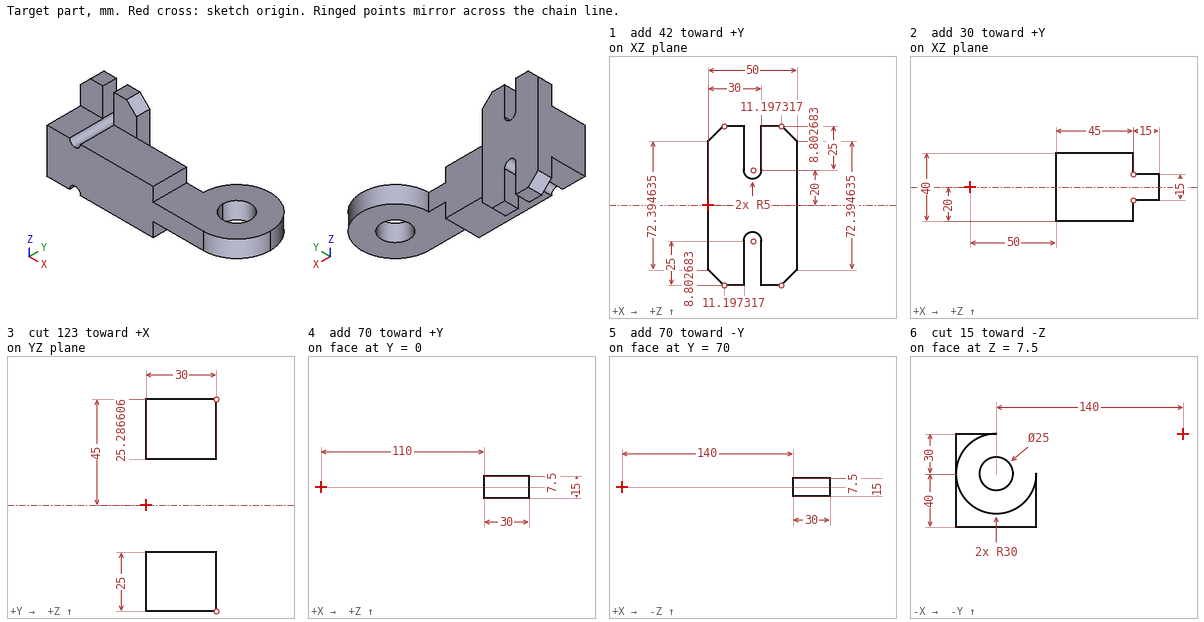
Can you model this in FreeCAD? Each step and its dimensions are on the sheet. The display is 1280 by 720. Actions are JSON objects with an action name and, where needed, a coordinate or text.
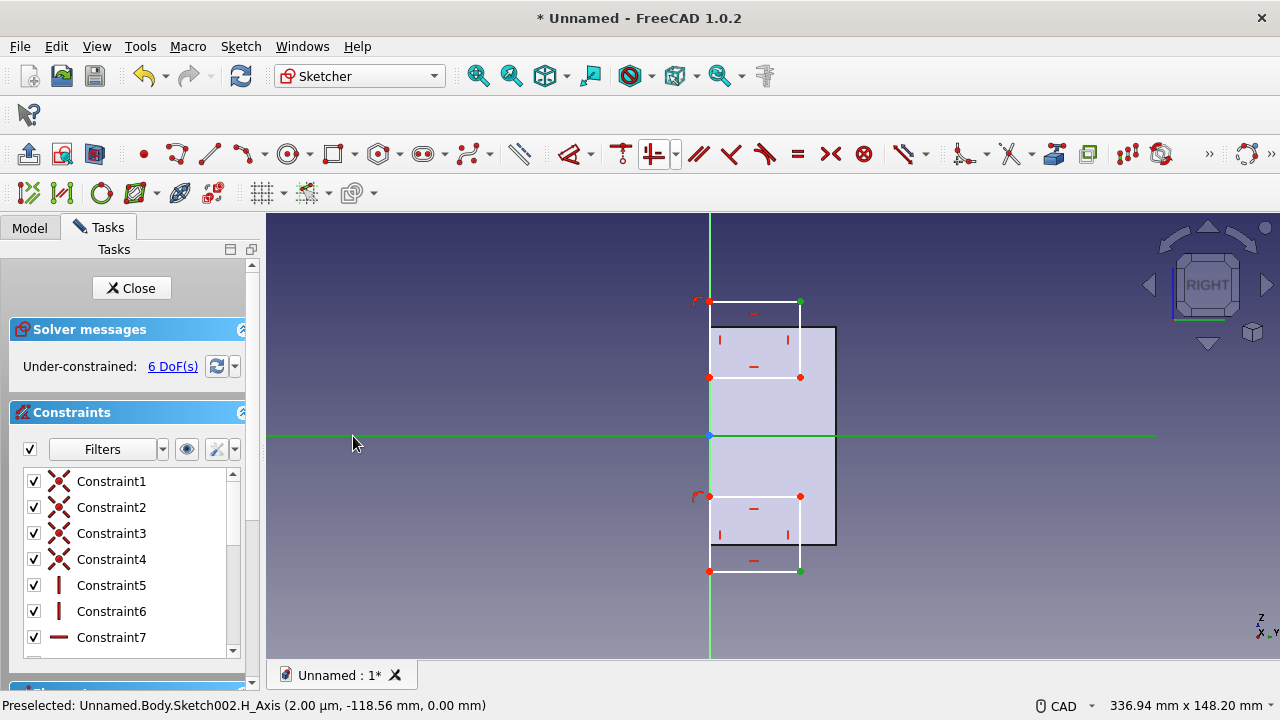
{"action": "left_click", "coordinate": [831, 154]}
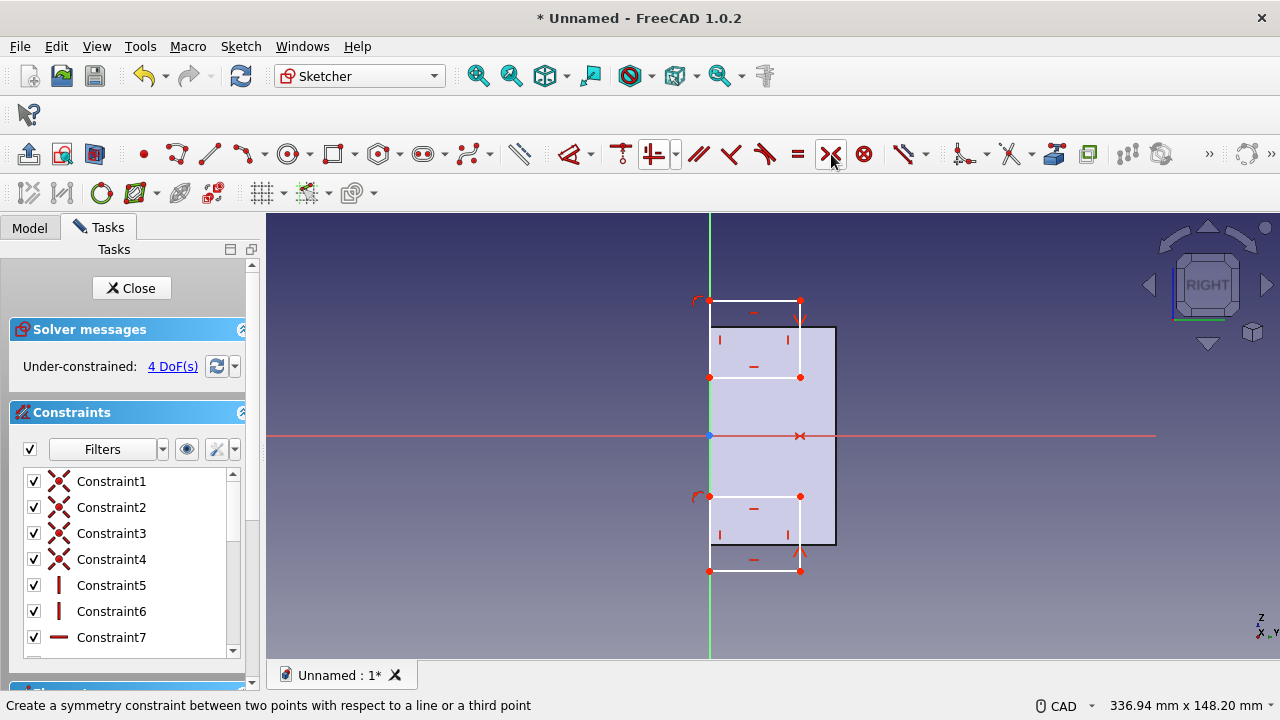
{"action": "left_click", "coordinate": [568, 154]}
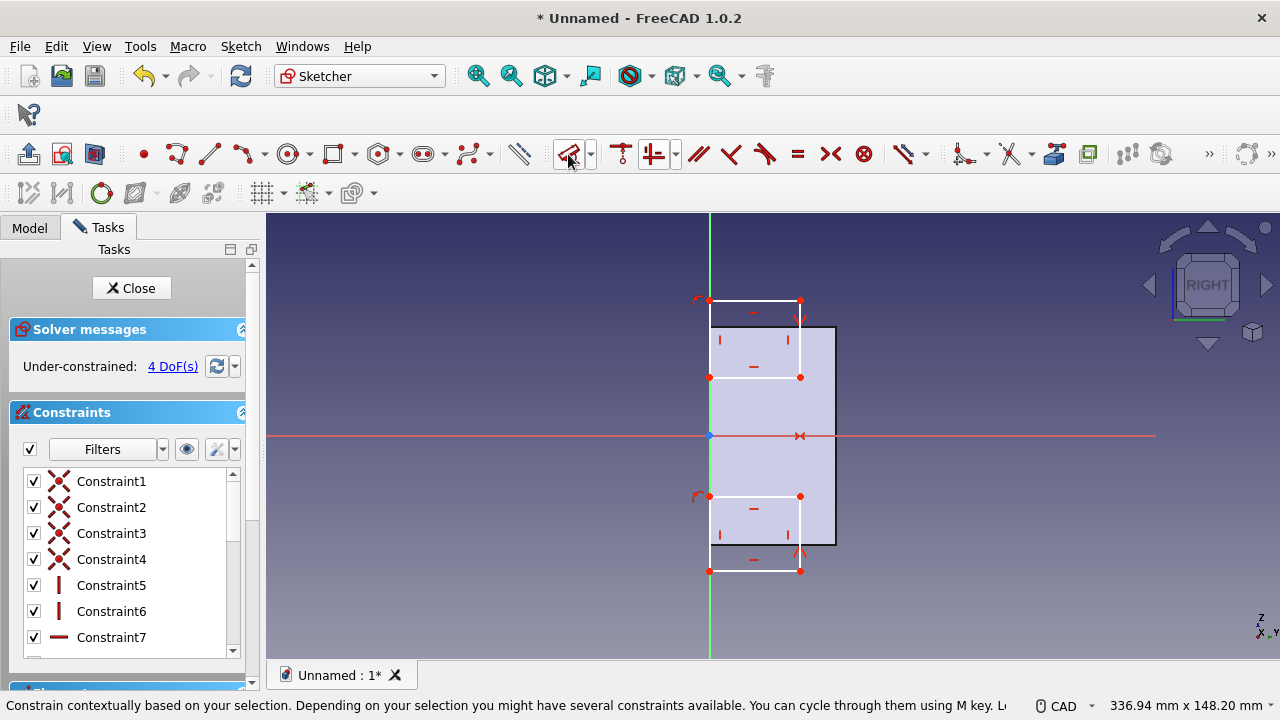
{"action": "left_click", "coordinate": [737, 378]}
{"action": "left_click", "coordinate": [755, 344]}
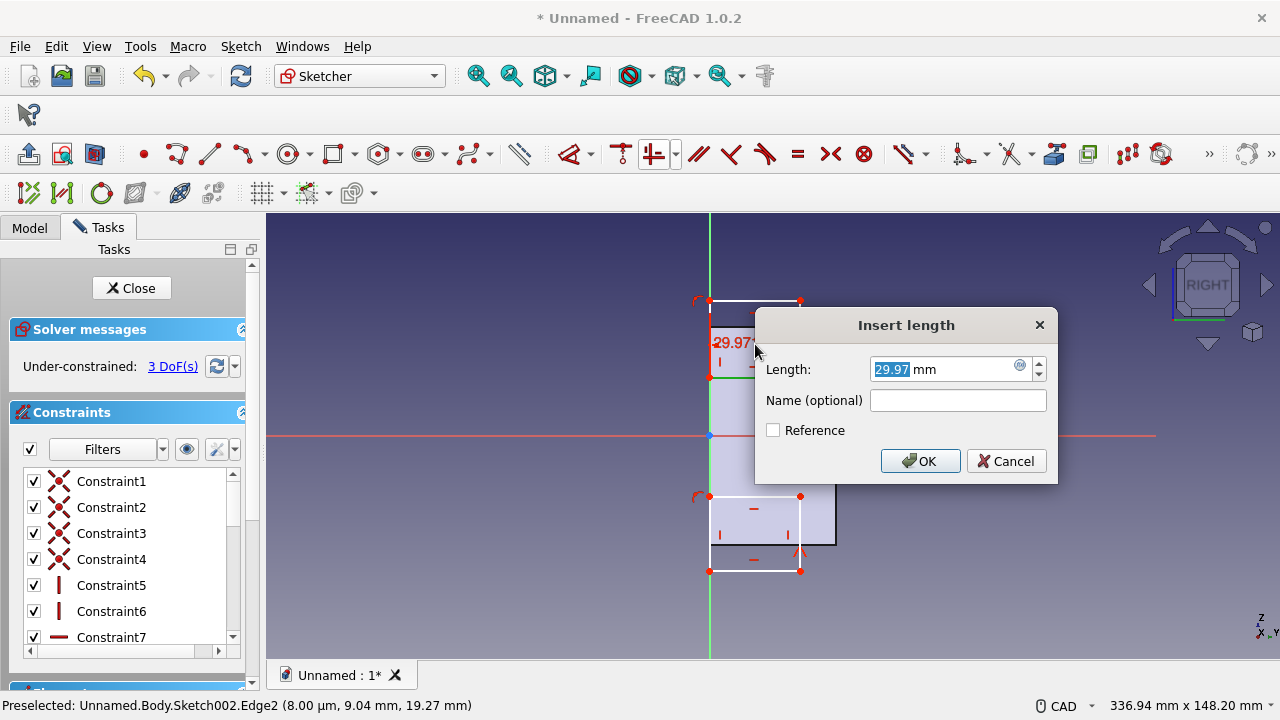
{"action": "type", "text": "30"}
{"action": "key", "text": "Return"}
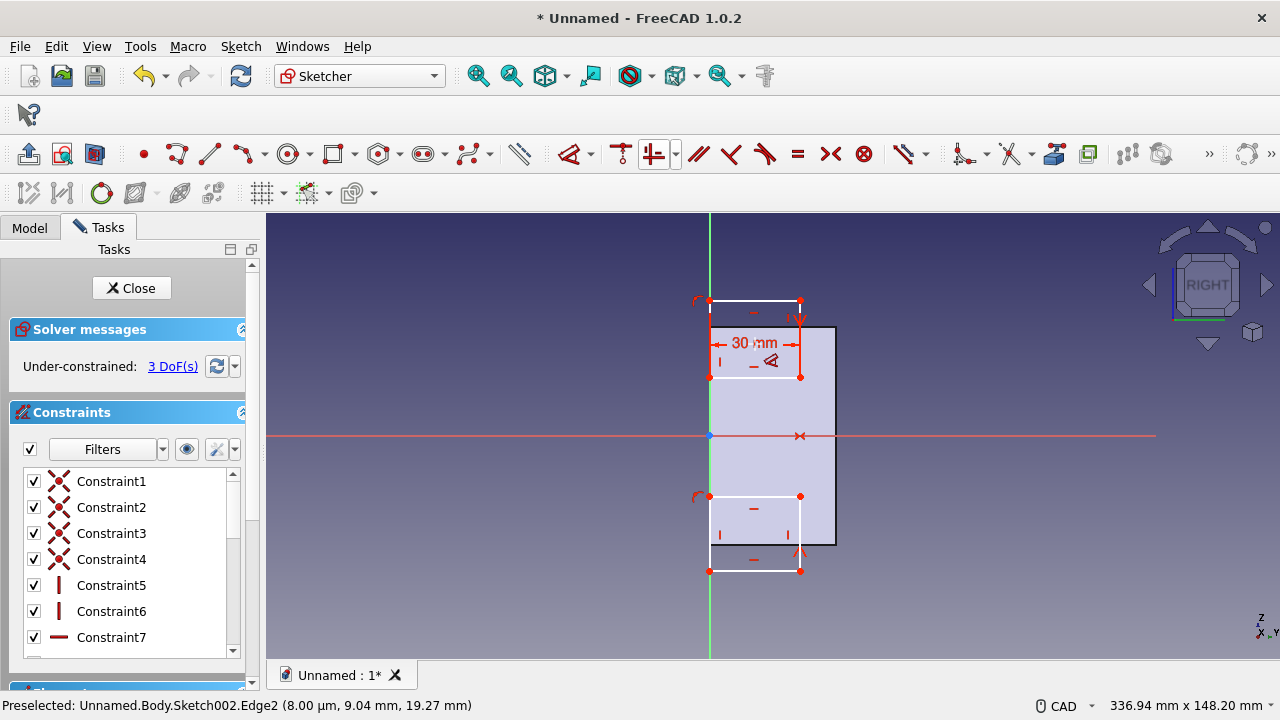
{"action": "left_click", "coordinate": [710, 519]}
{"action": "left_click", "coordinate": [676, 534]}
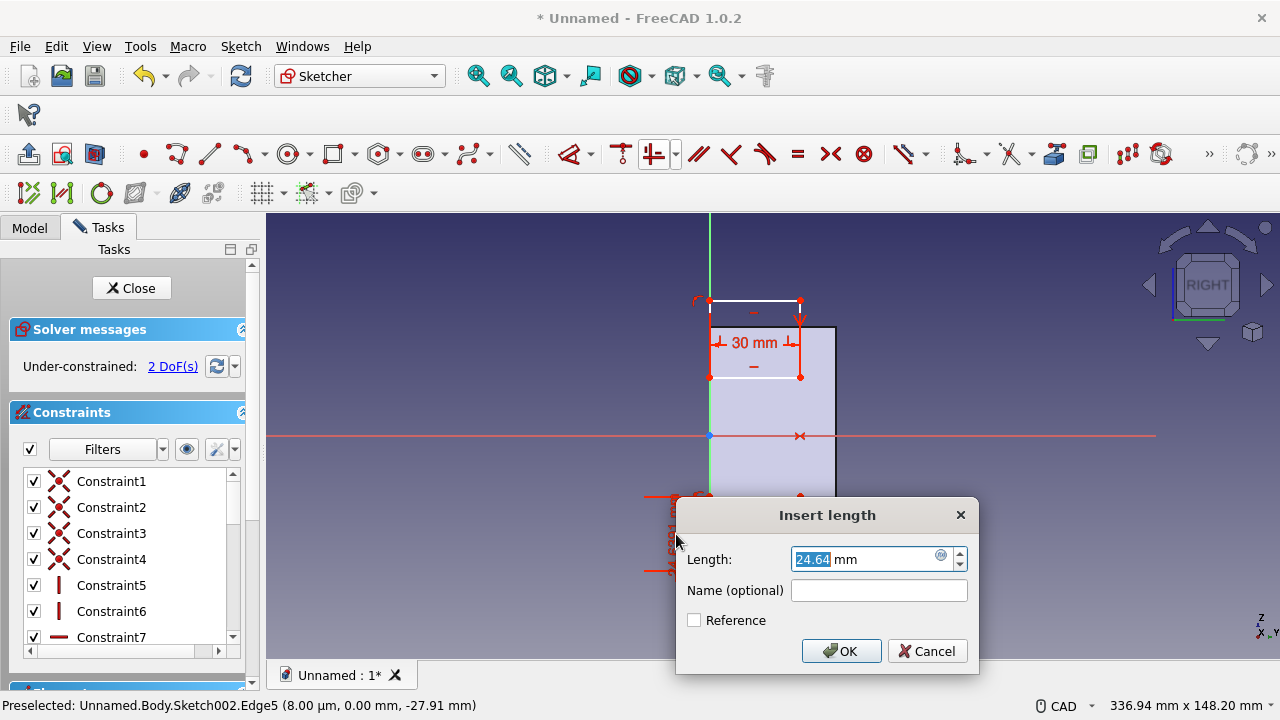
{"action": "type", "text": "25"}
{"action": "key", "text": "Return"}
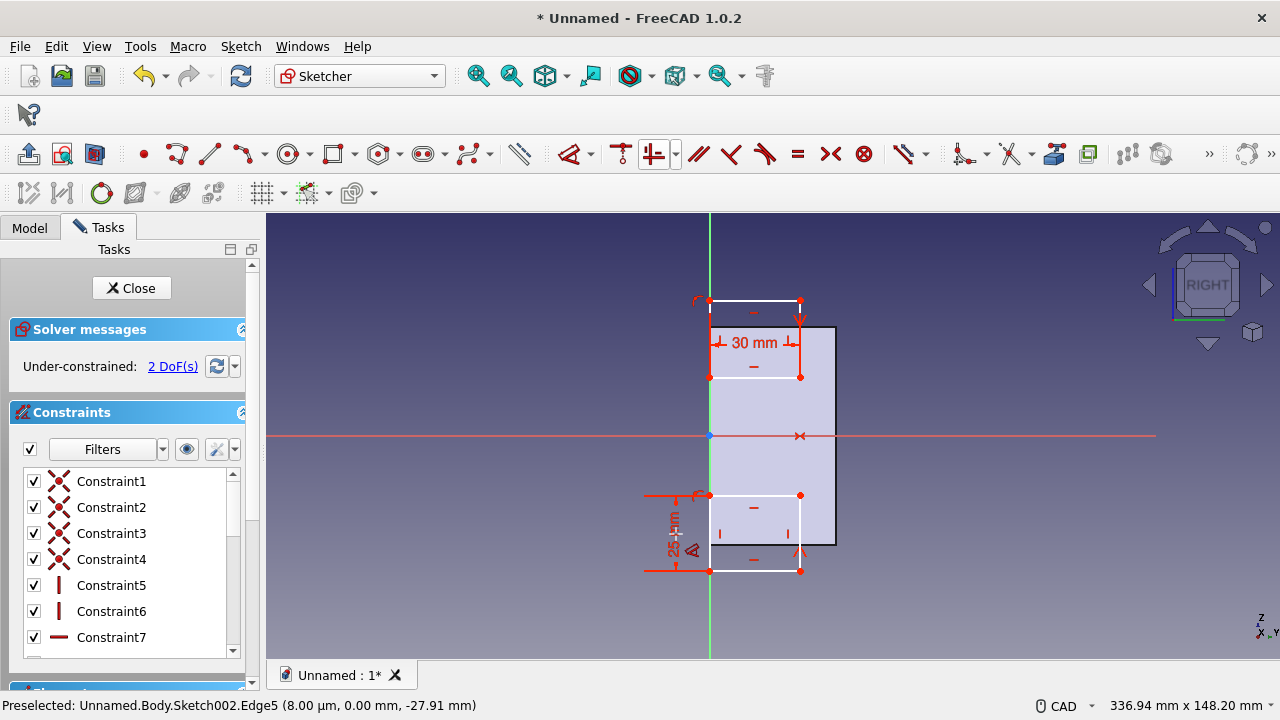
{"action": "left_click", "coordinate": [710, 301]}
{"action": "left_click", "coordinate": [676, 368]}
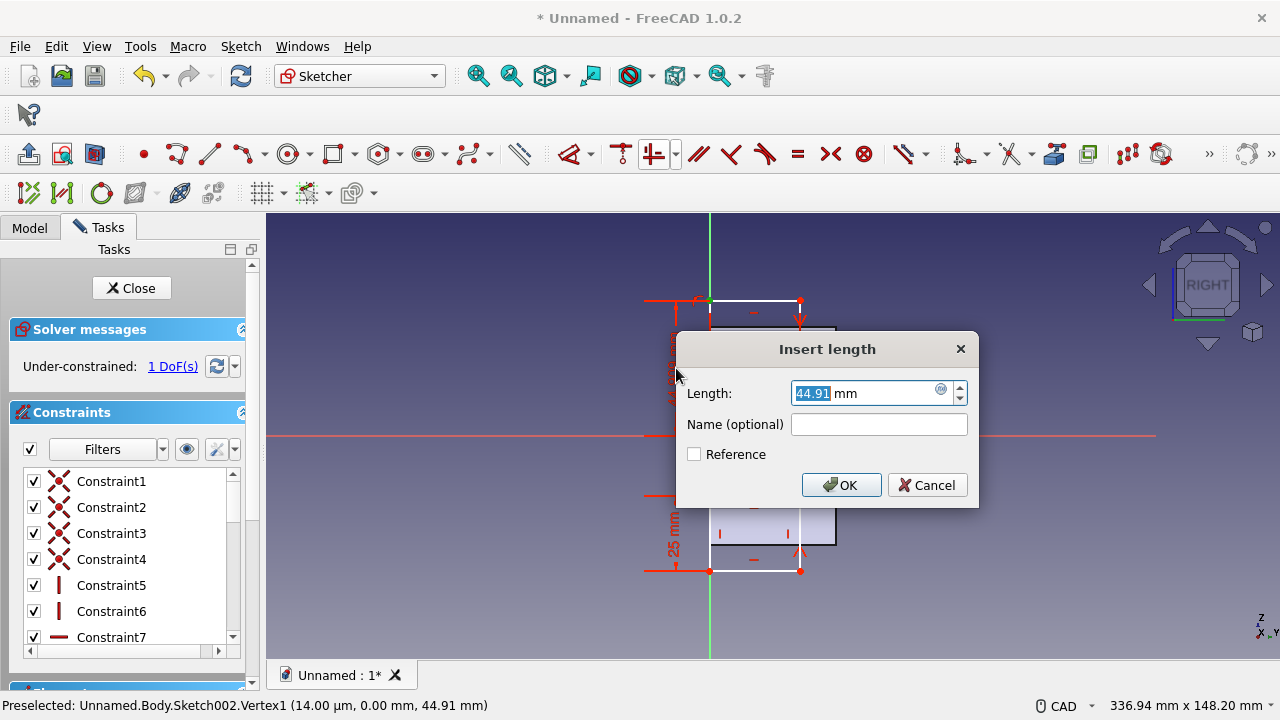
{"action": "type", "text": "45"}
{"action": "key", "text": "Return"}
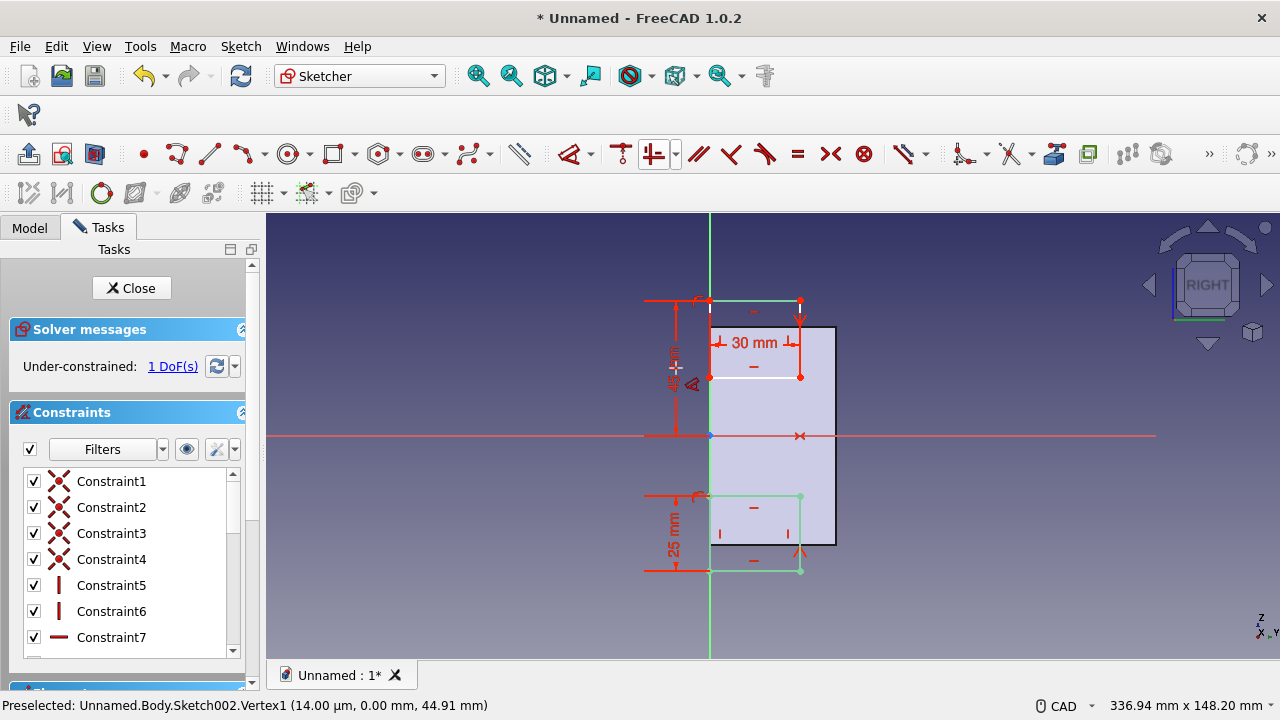
{"action": "left_click", "coordinate": [710, 324]}
{"action": "left_click", "coordinate": [676, 339]}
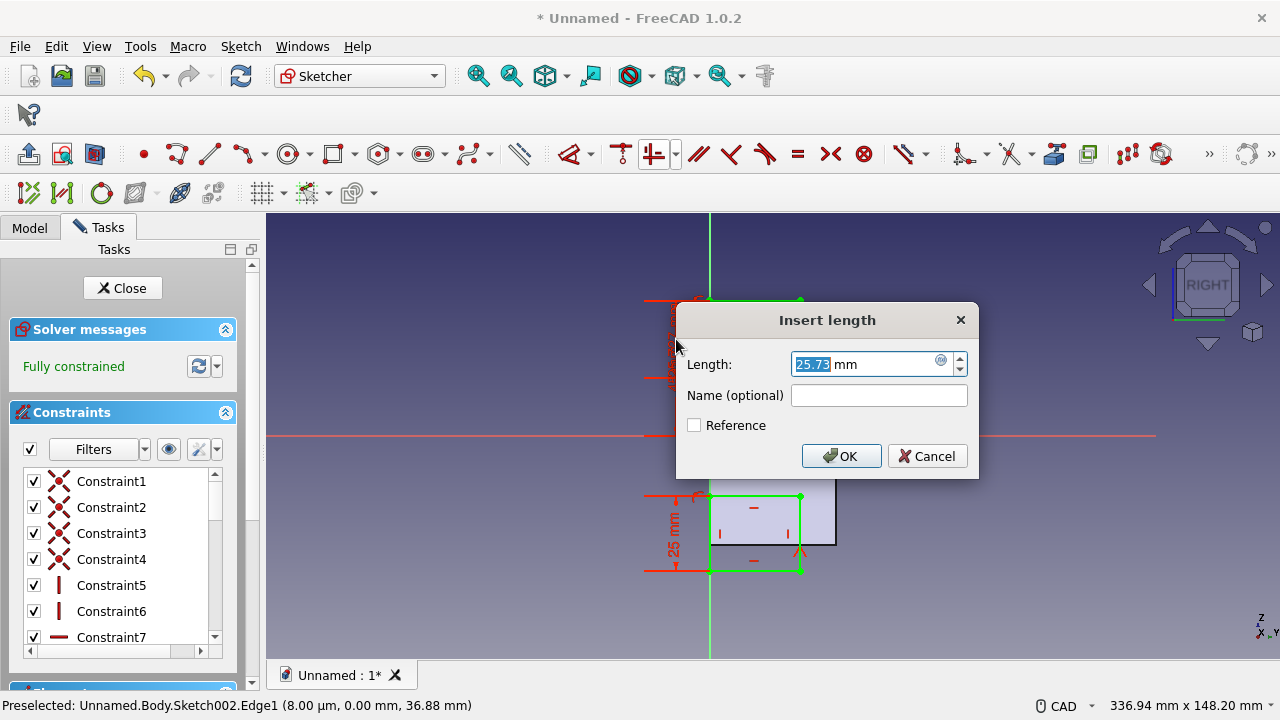
{"action": "type", "text": "25.286606"}
{"action": "key", "text": "Return"}
{"action": "key", "text": "Escape"}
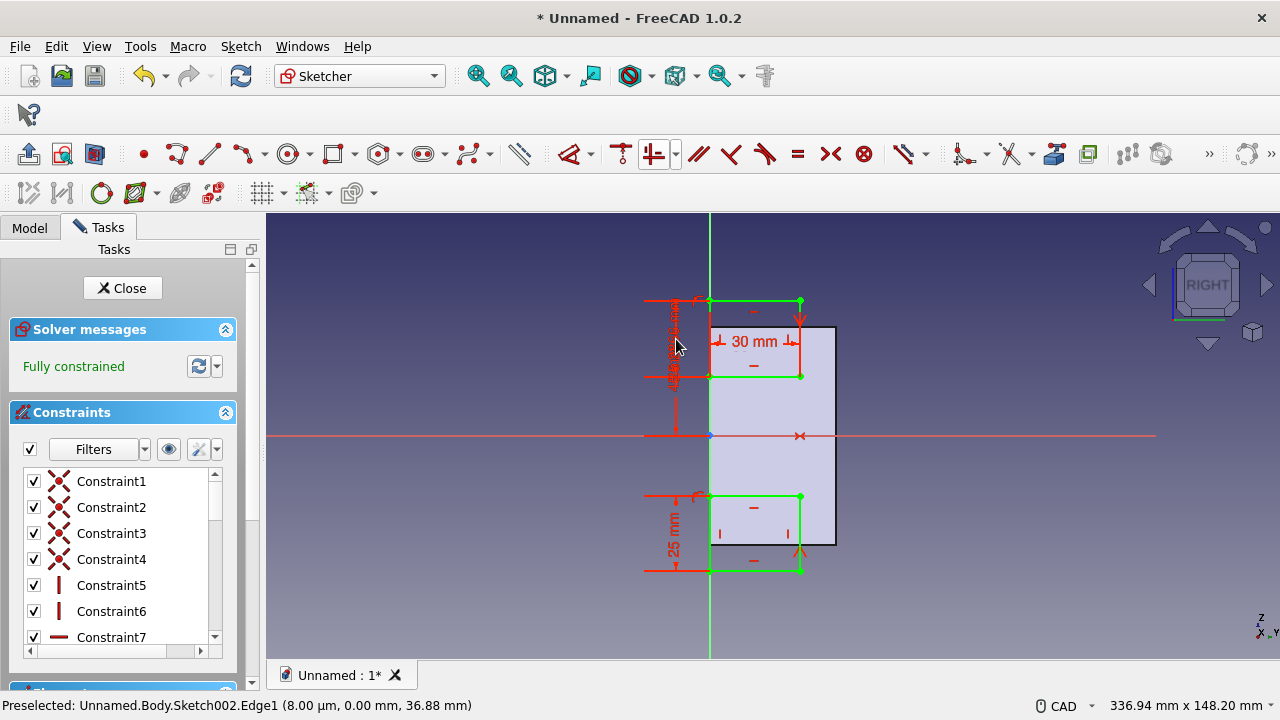
{"action": "left_click", "coordinate": [123, 288]}